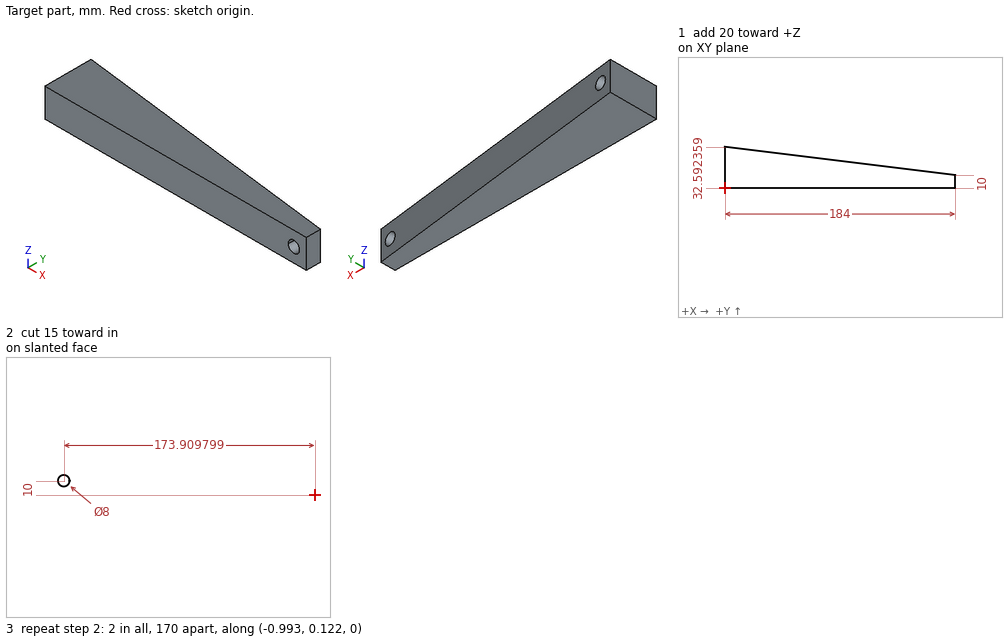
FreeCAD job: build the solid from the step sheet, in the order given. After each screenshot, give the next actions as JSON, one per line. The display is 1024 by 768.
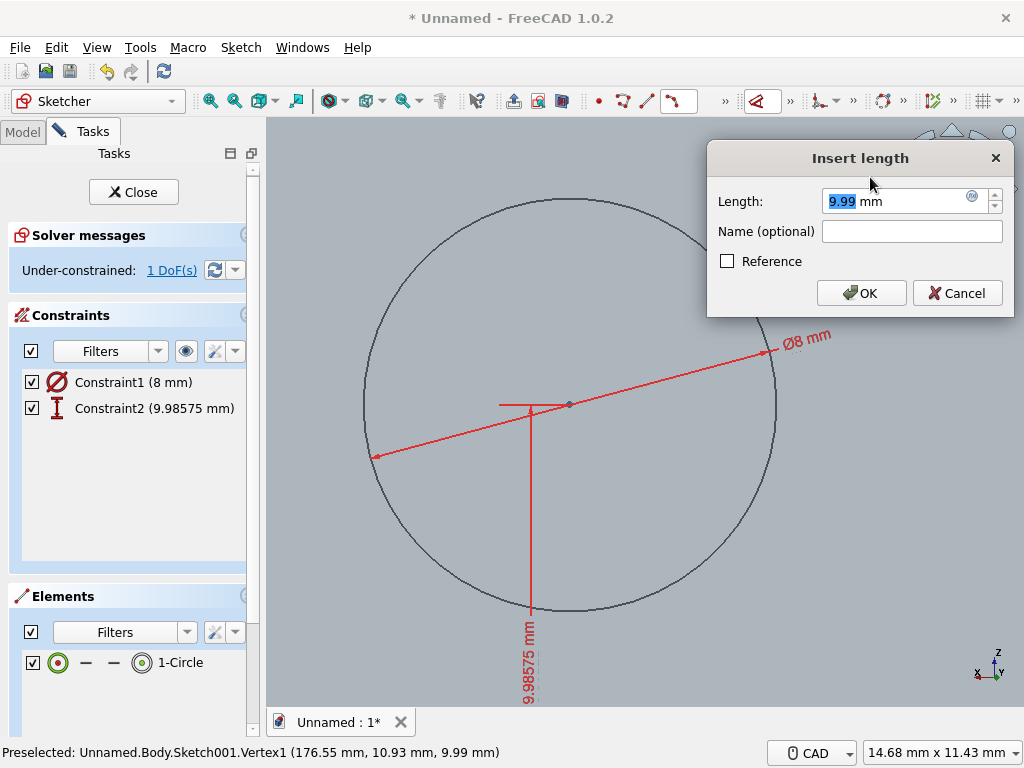
{"action": "type", "text": "10"}
{"action": "key", "text": "Return"}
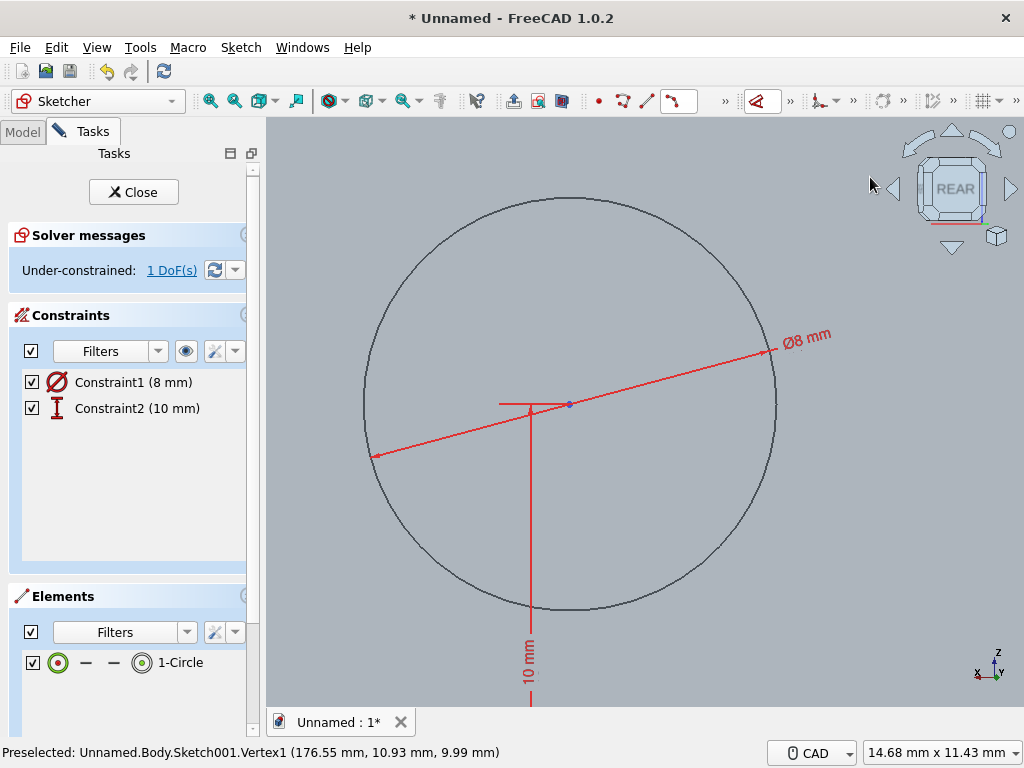
{"action": "left_click", "coordinate": [570, 404]}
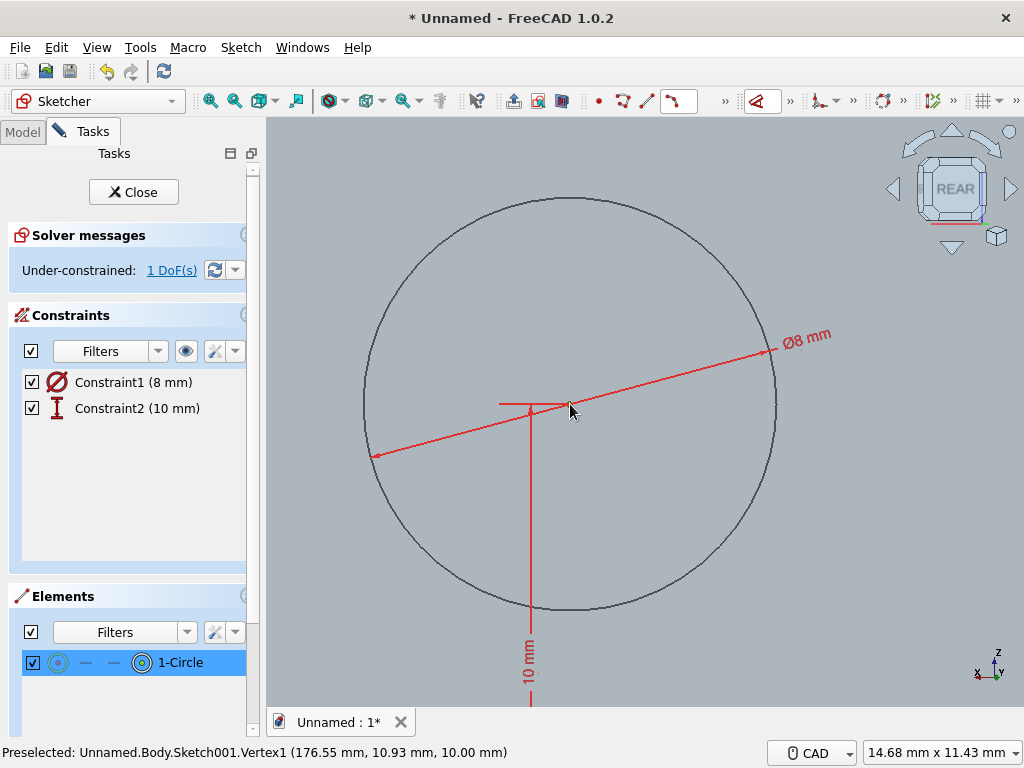
{"action": "key", "text": "l"}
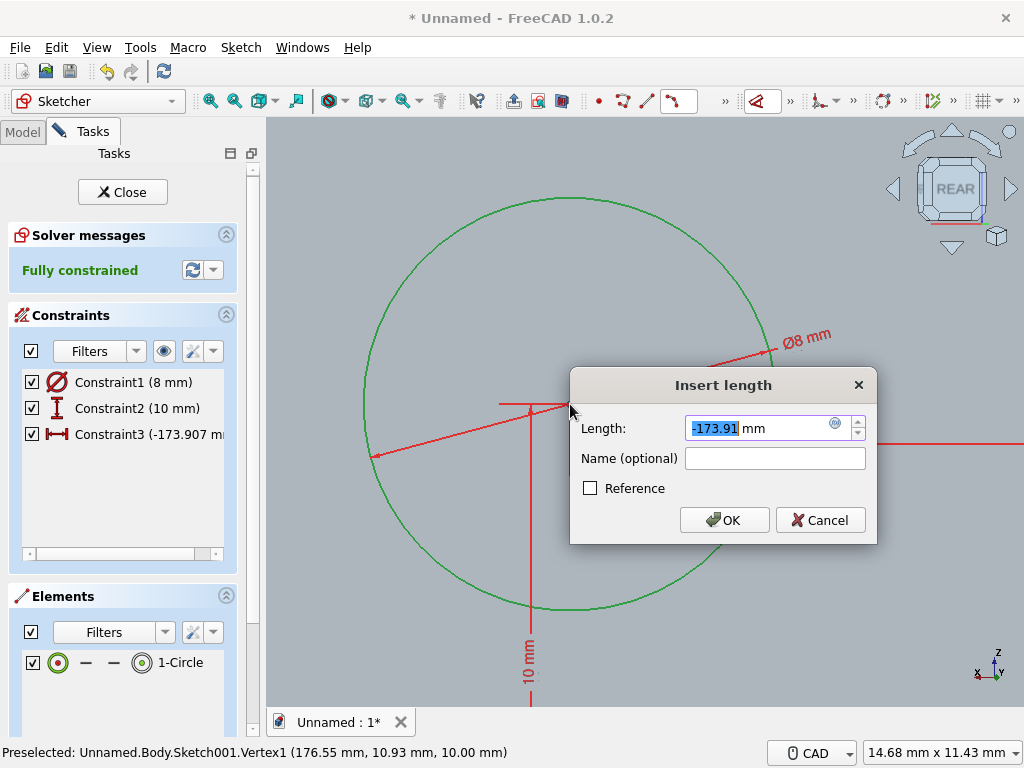
{"action": "type", "text": "-173.909799"}
{"action": "key", "text": "Return"}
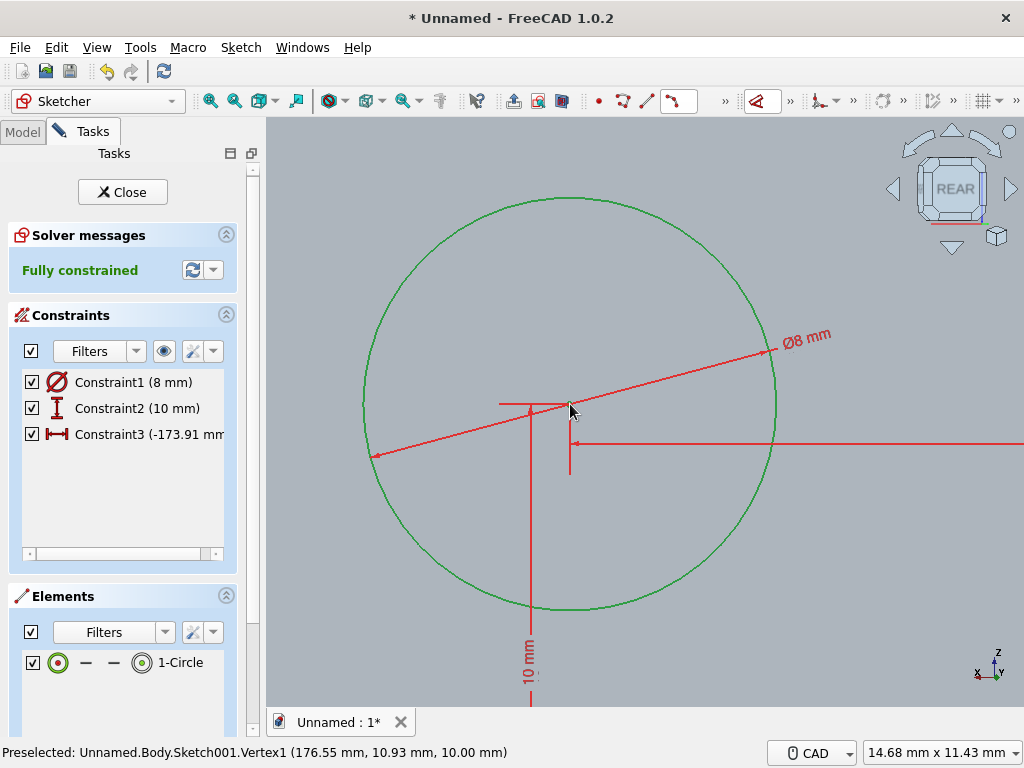
{"action": "left_click", "coordinate": [123, 192]}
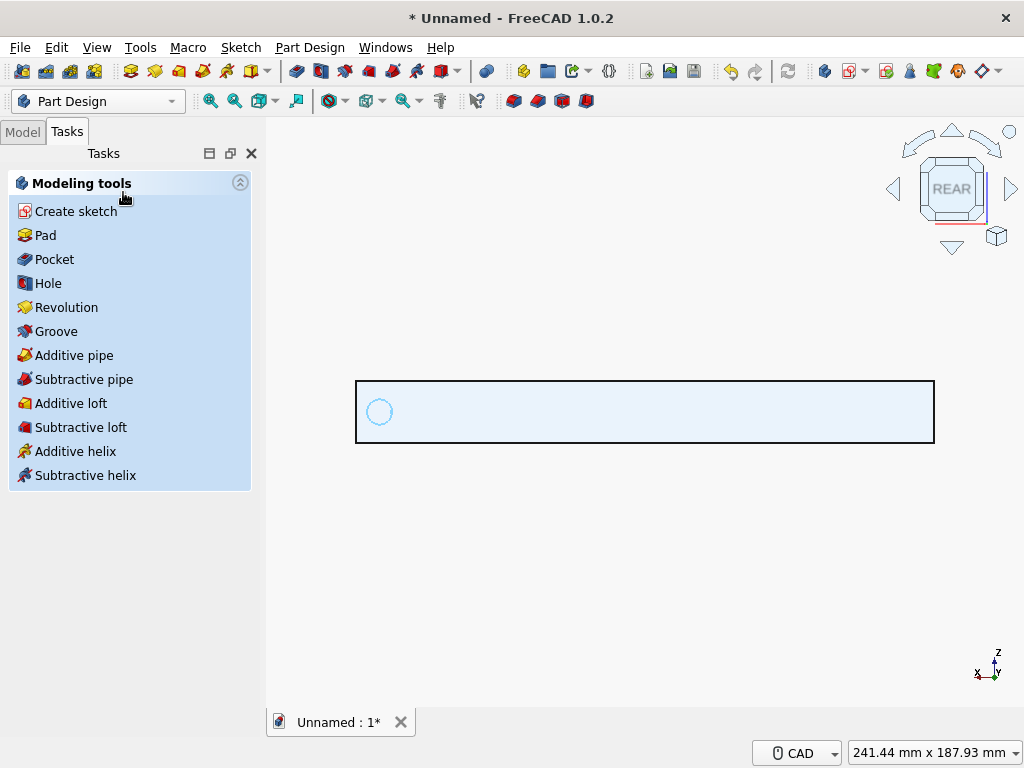
{"action": "left_click", "coordinate": [298, 72]}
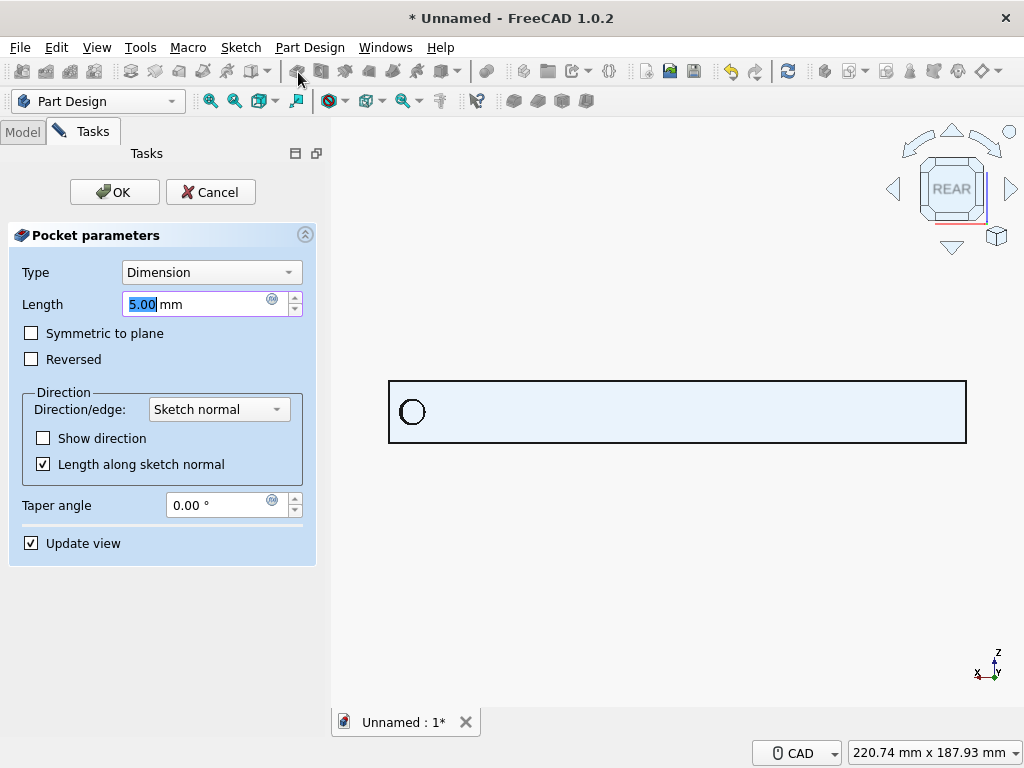
{"action": "type", "text": "15"}
{"action": "key", "text": "Tab"}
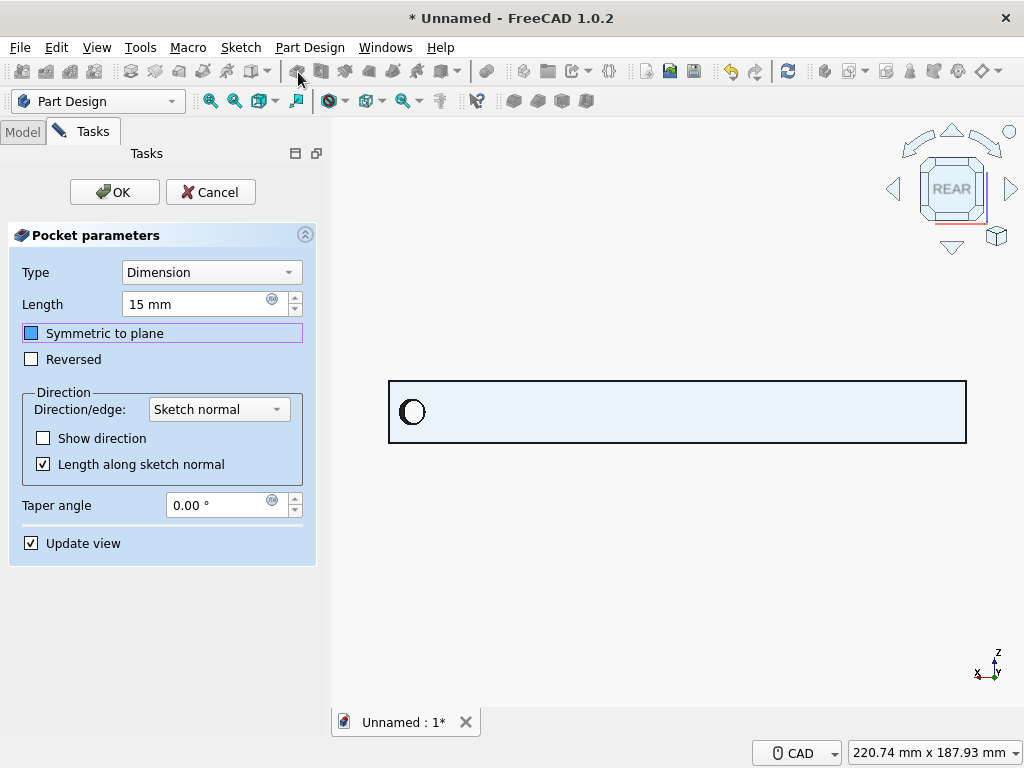
{"action": "left_click", "coordinate": [115, 192]}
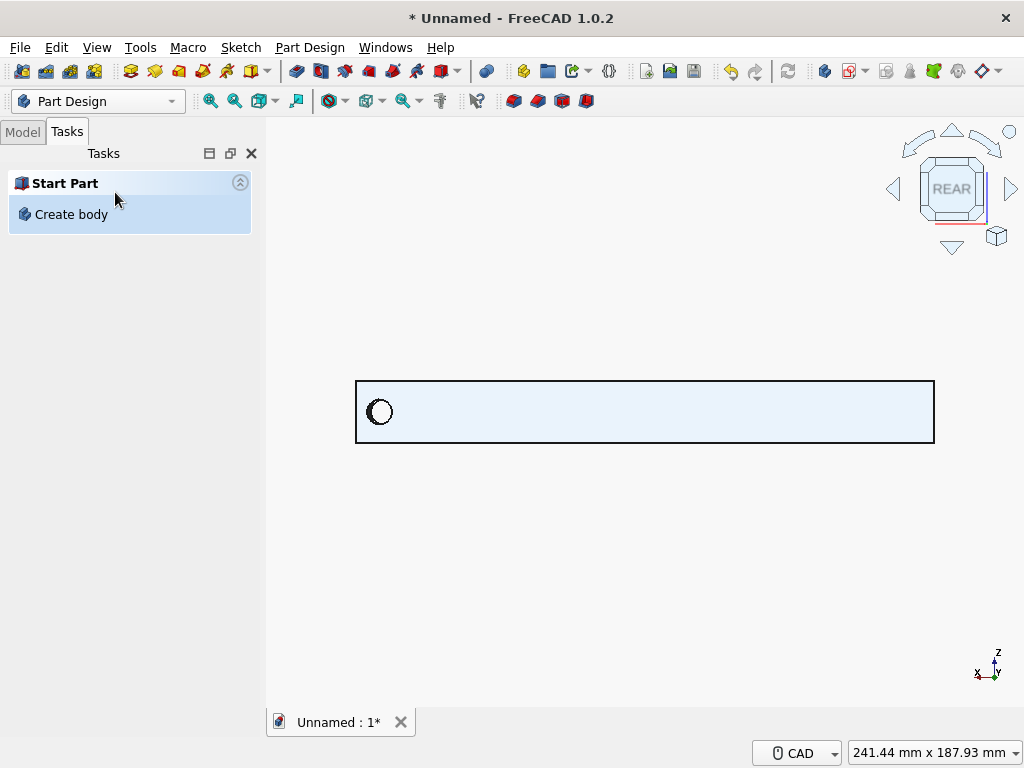
{"action": "left_click", "coordinate": [23, 131]}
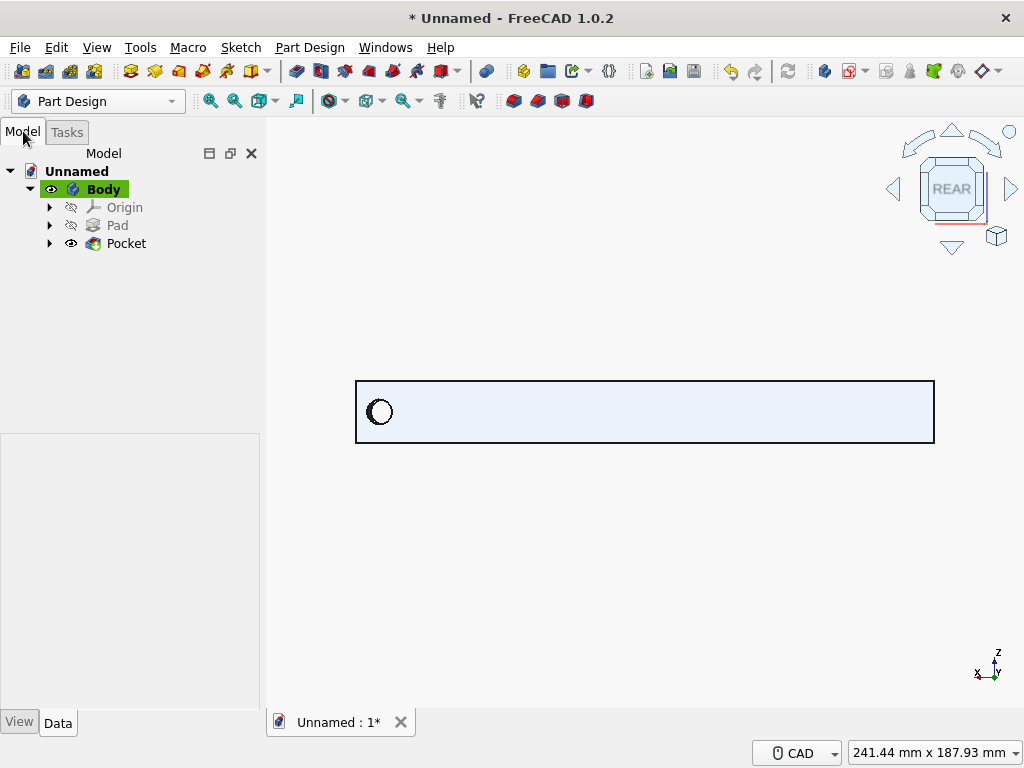
{"action": "left_click", "coordinate": [116, 243]}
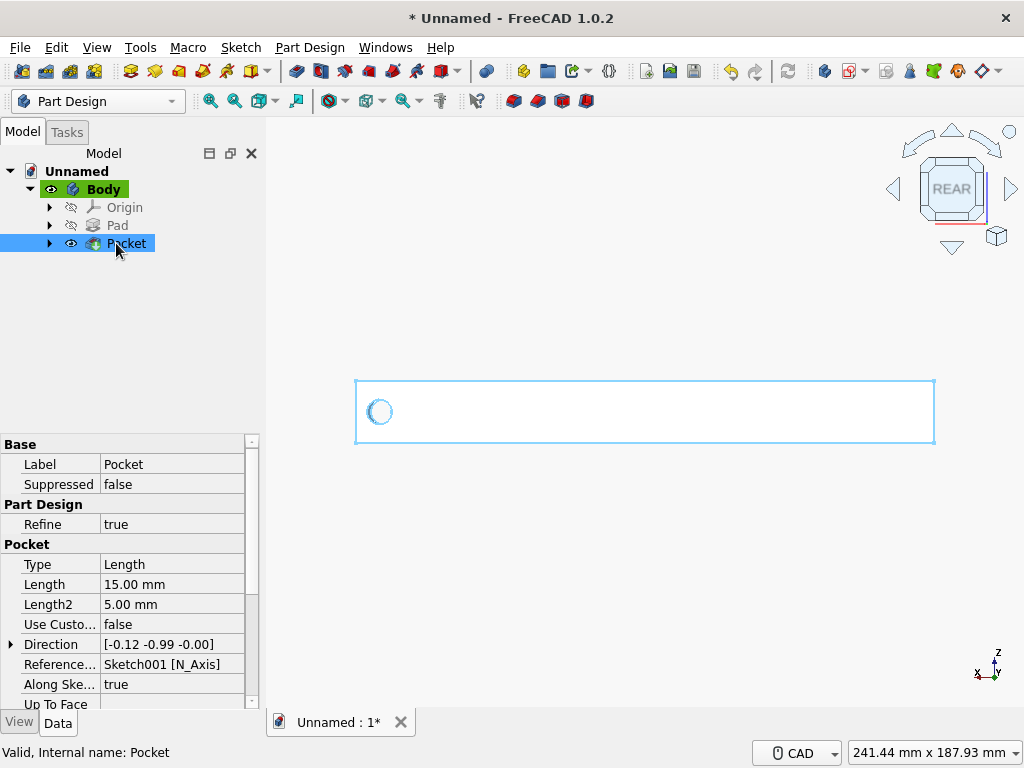
{"action": "left_click", "coordinate": [46, 72]}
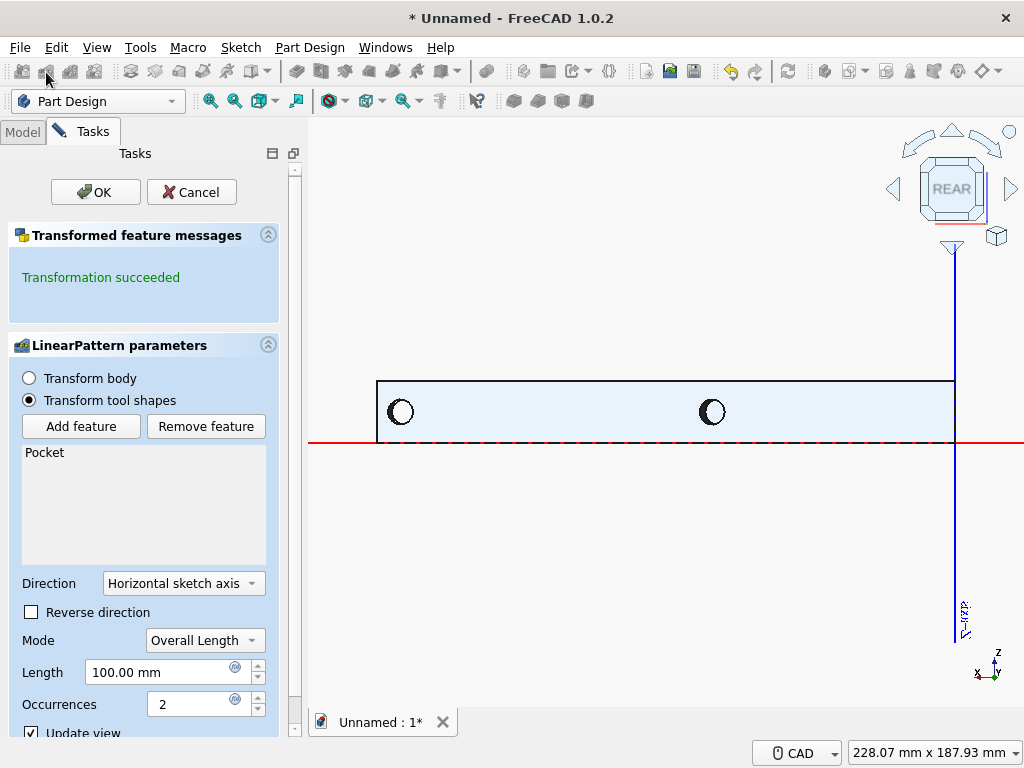
{"action": "left_click", "coordinate": [206, 640]}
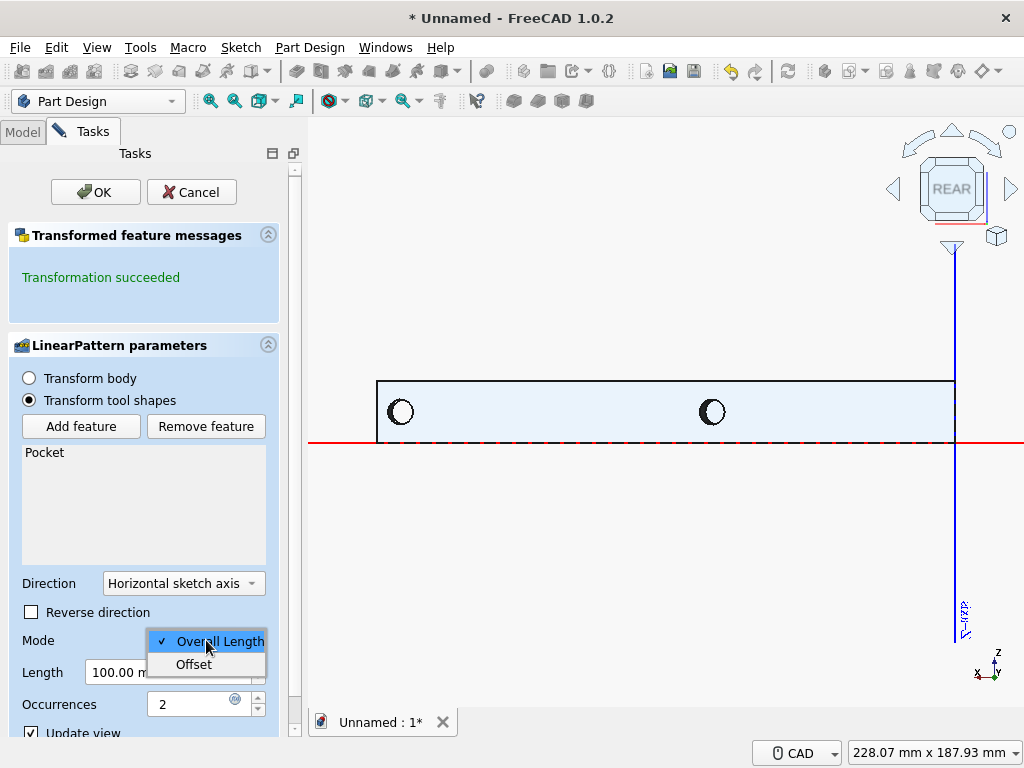
{"action": "left_click", "coordinate": [206, 664]}